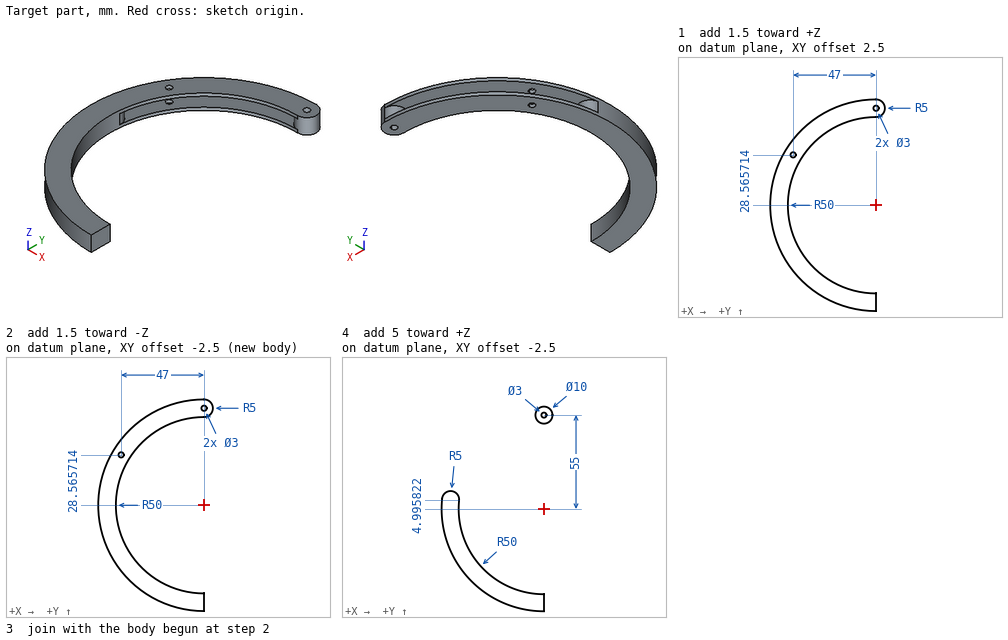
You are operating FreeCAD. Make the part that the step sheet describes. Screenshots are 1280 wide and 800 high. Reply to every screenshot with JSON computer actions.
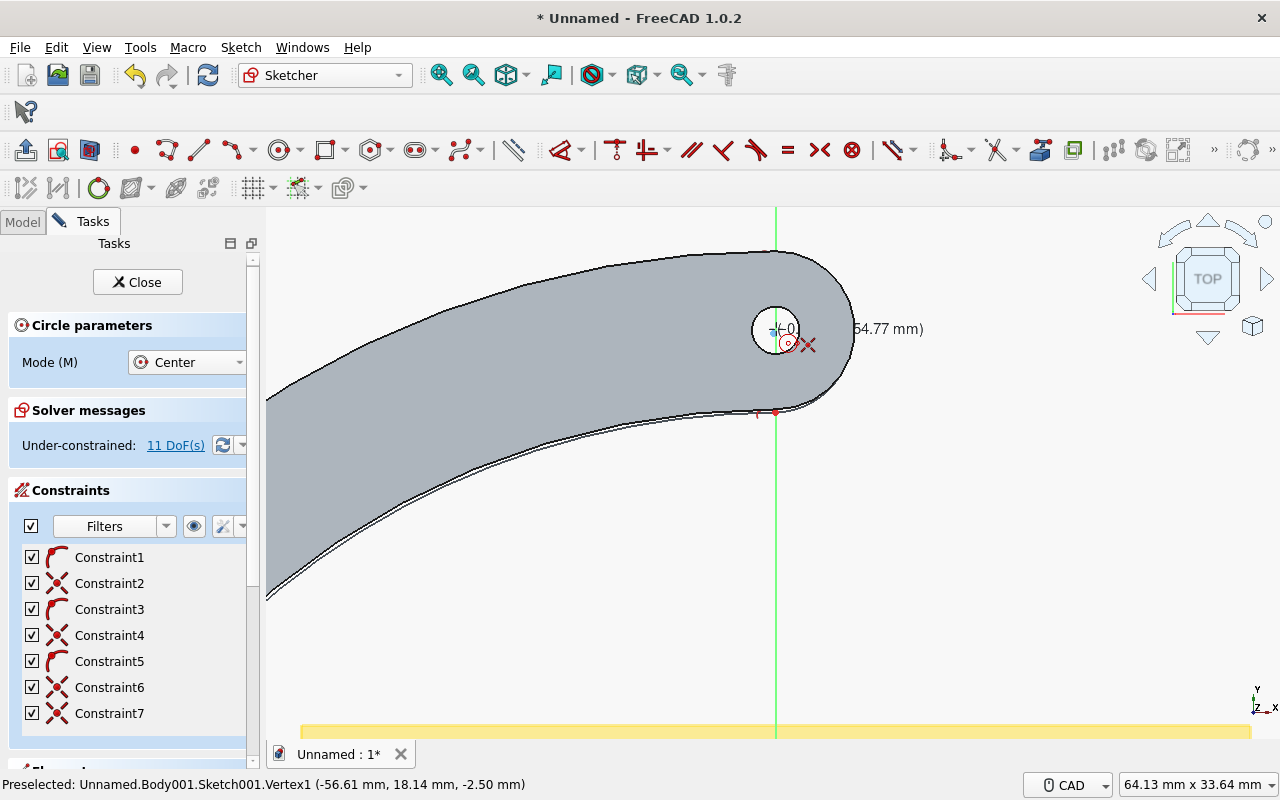
{"action": "scroll", "coordinate": [777, 329], "scroll_direction": "down", "scroll_amount": 9}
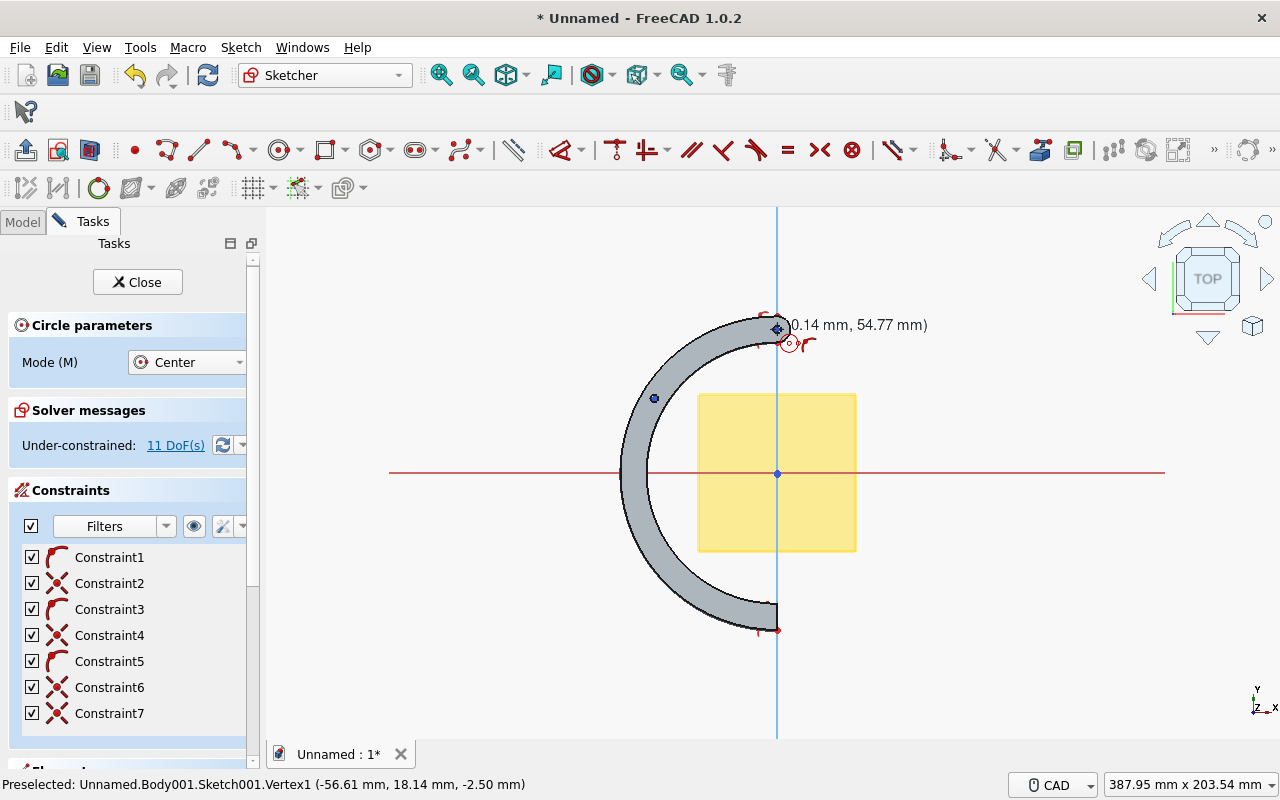
{"action": "left_click", "coordinate": [777, 329]}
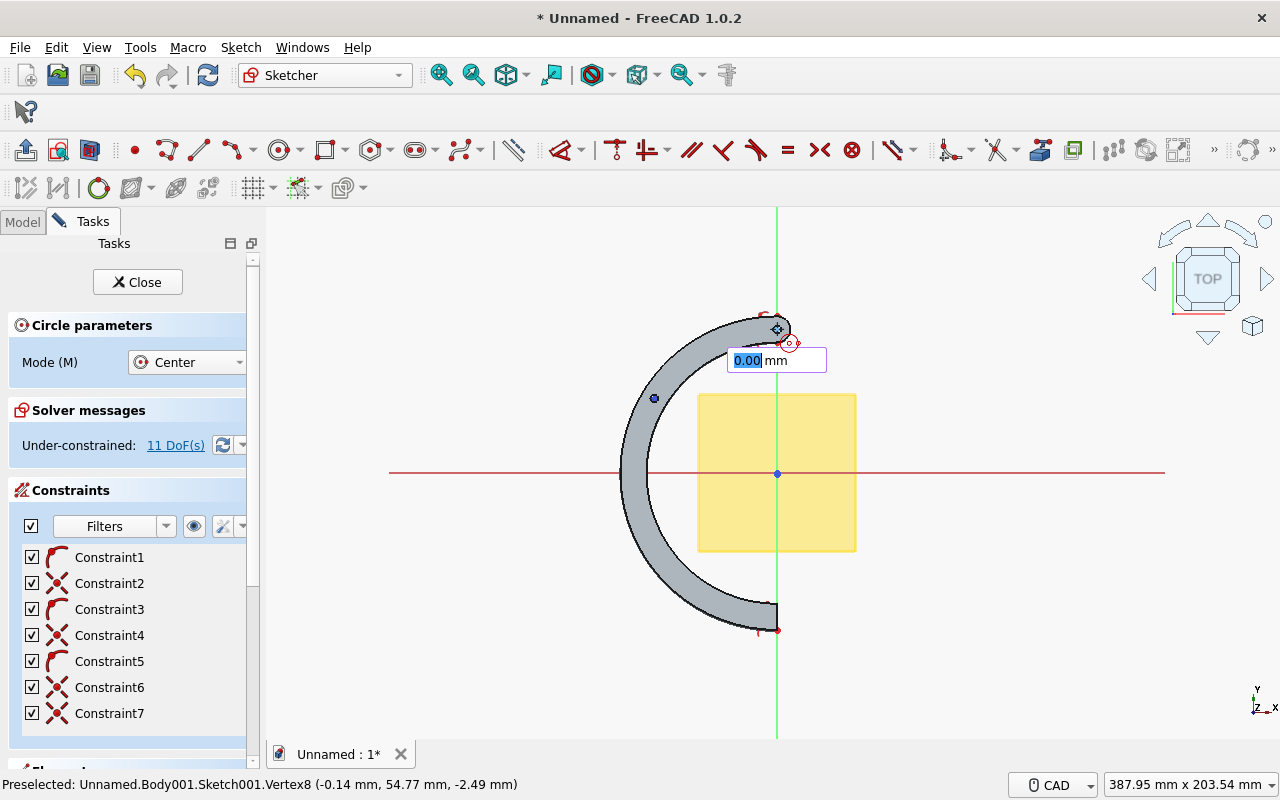
{"action": "scroll", "coordinate": [781, 328], "scroll_direction": "up", "scroll_amount": 8}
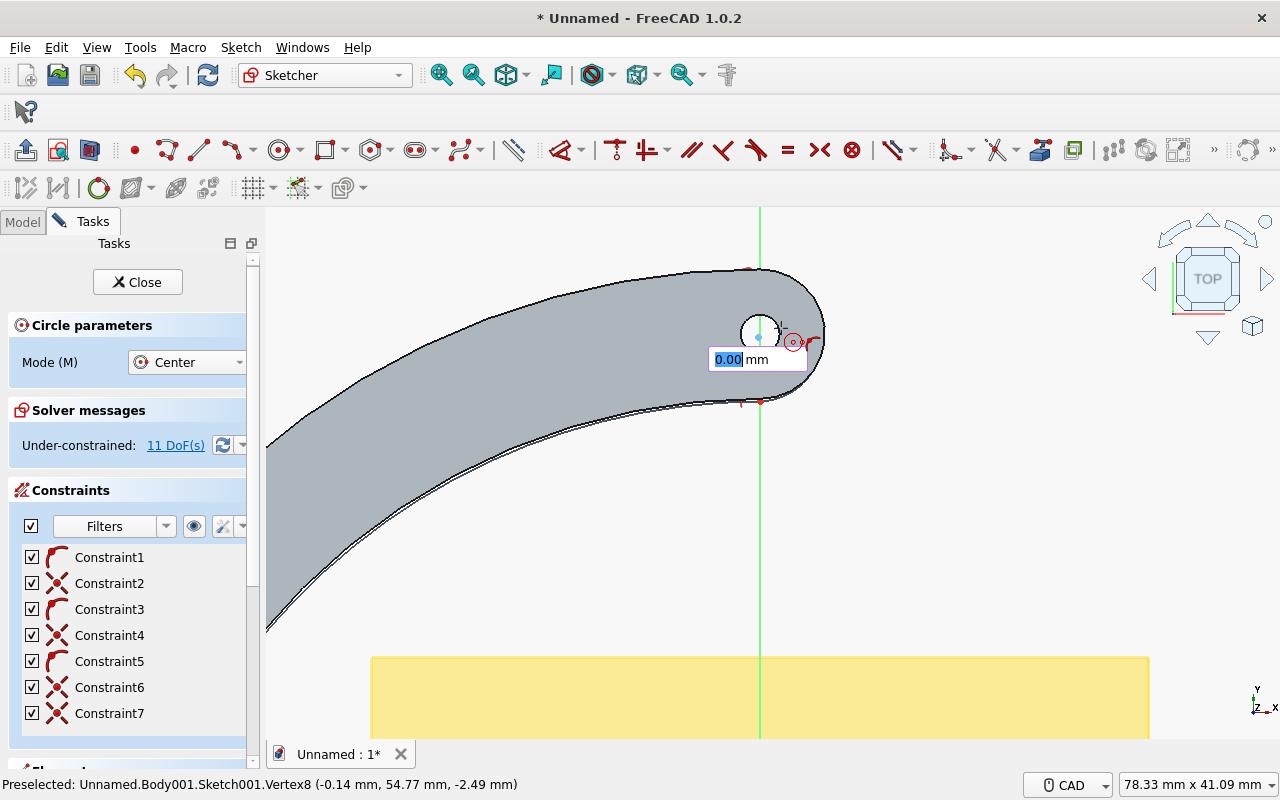
{"action": "left_click", "coordinate": [778, 327]}
{"action": "key", "text": "Escape"}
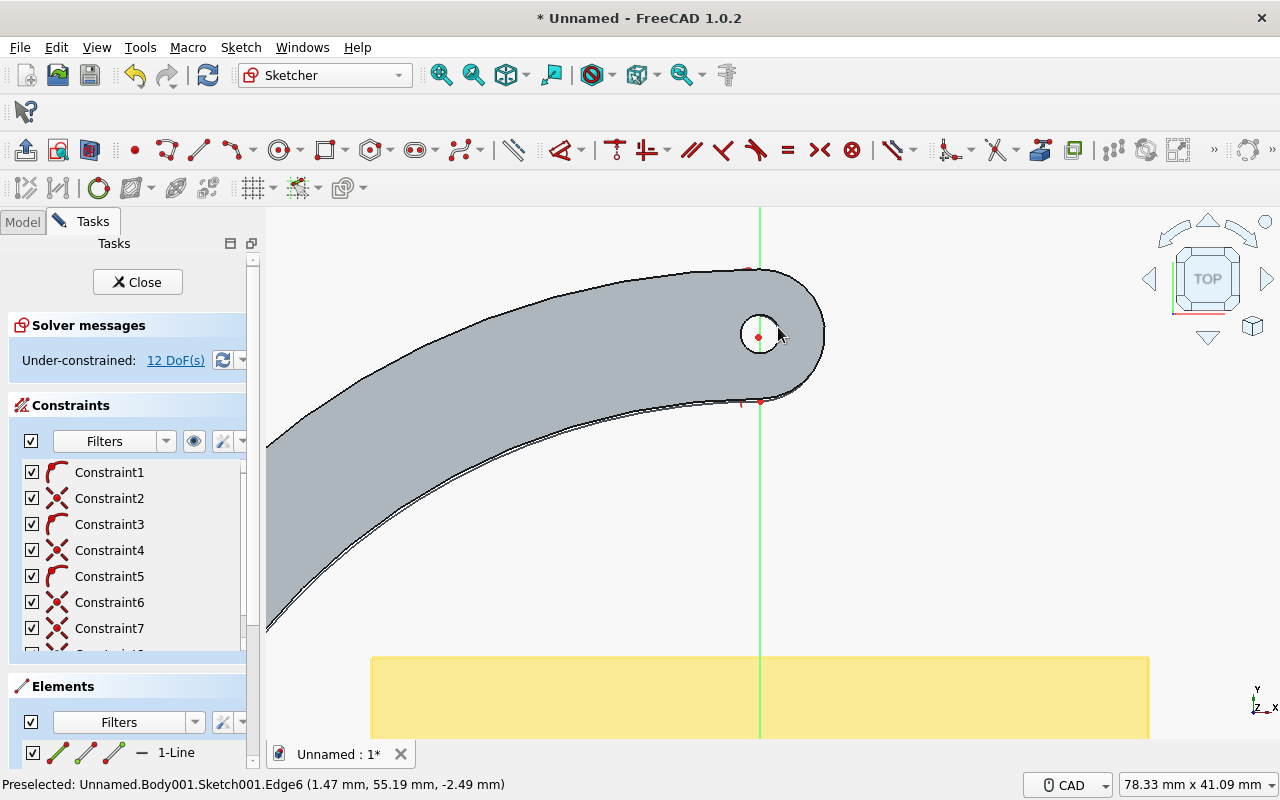
{"action": "scroll", "coordinate": [780, 328], "scroll_direction": "down", "scroll_amount": 8}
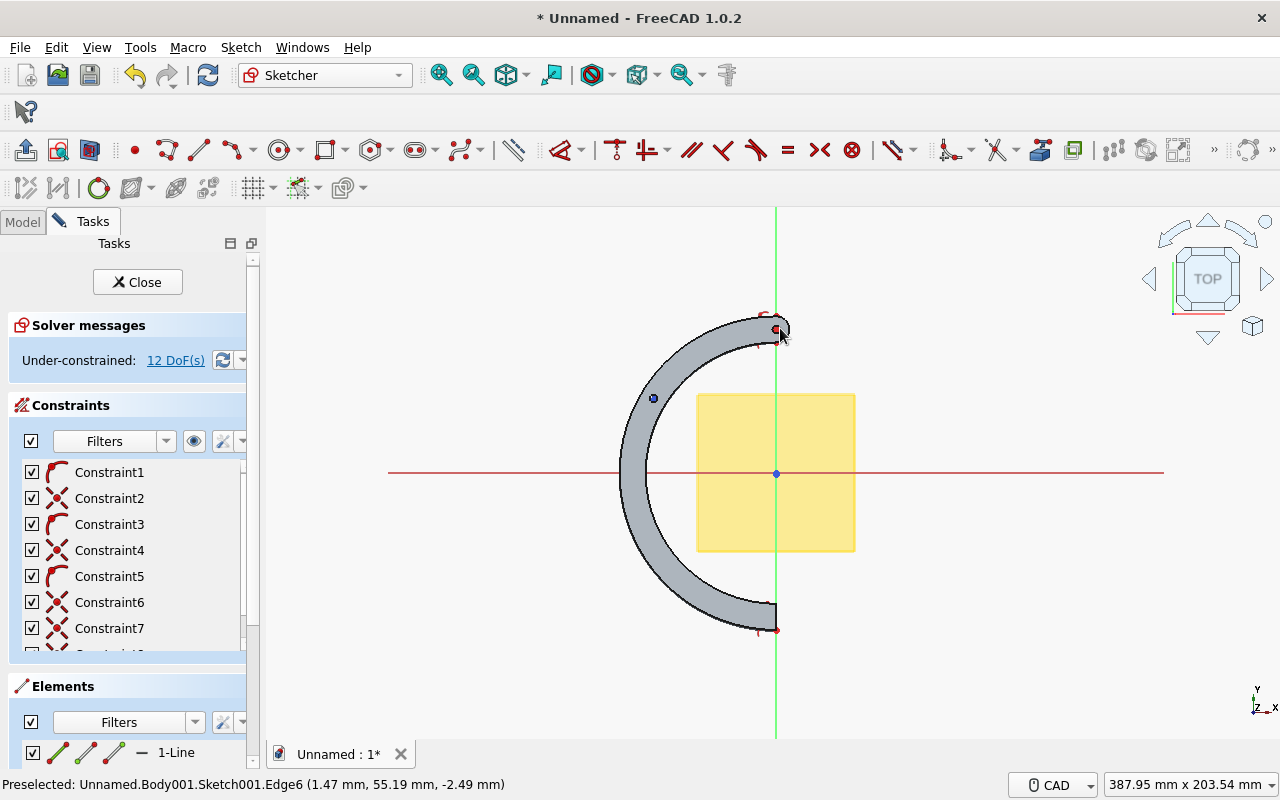
{"action": "left_click", "coordinate": [701, 367]}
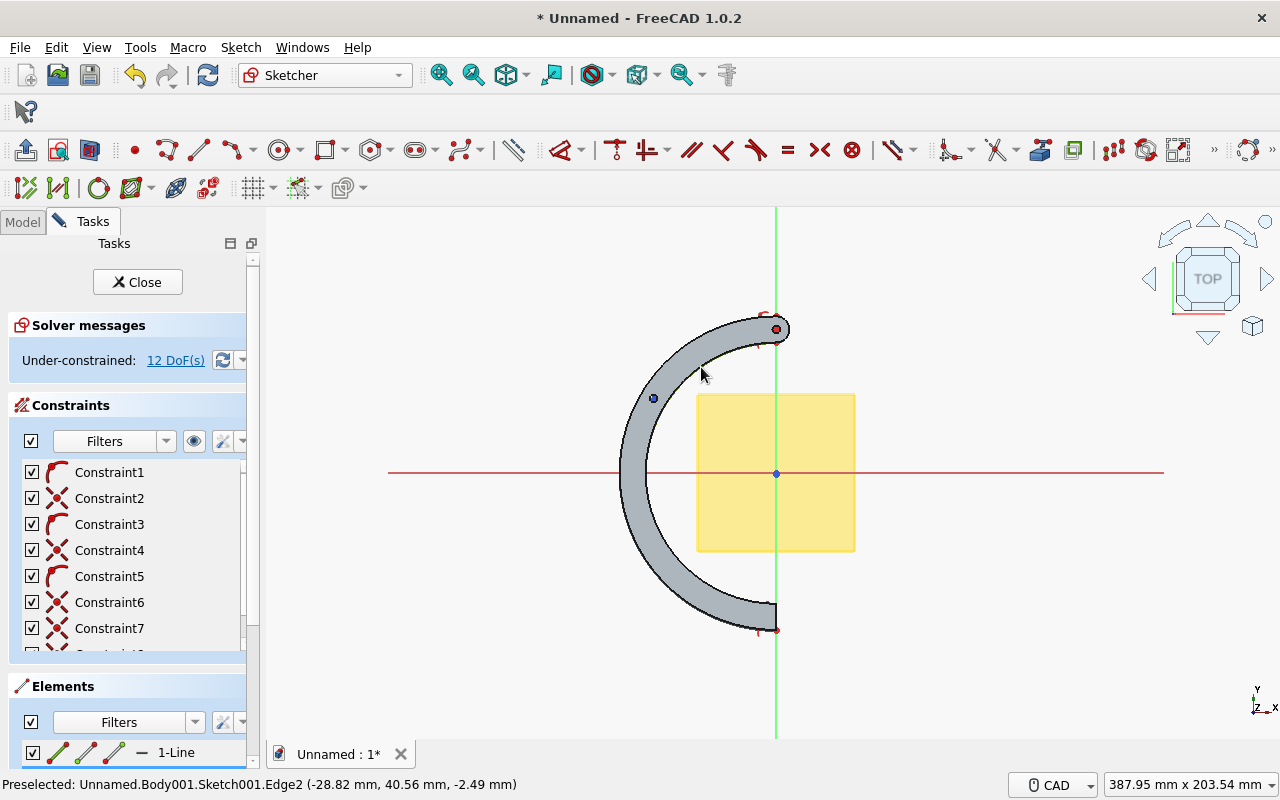
{"action": "scroll", "coordinate": [787, 338], "scroll_direction": "up", "scroll_amount": 3}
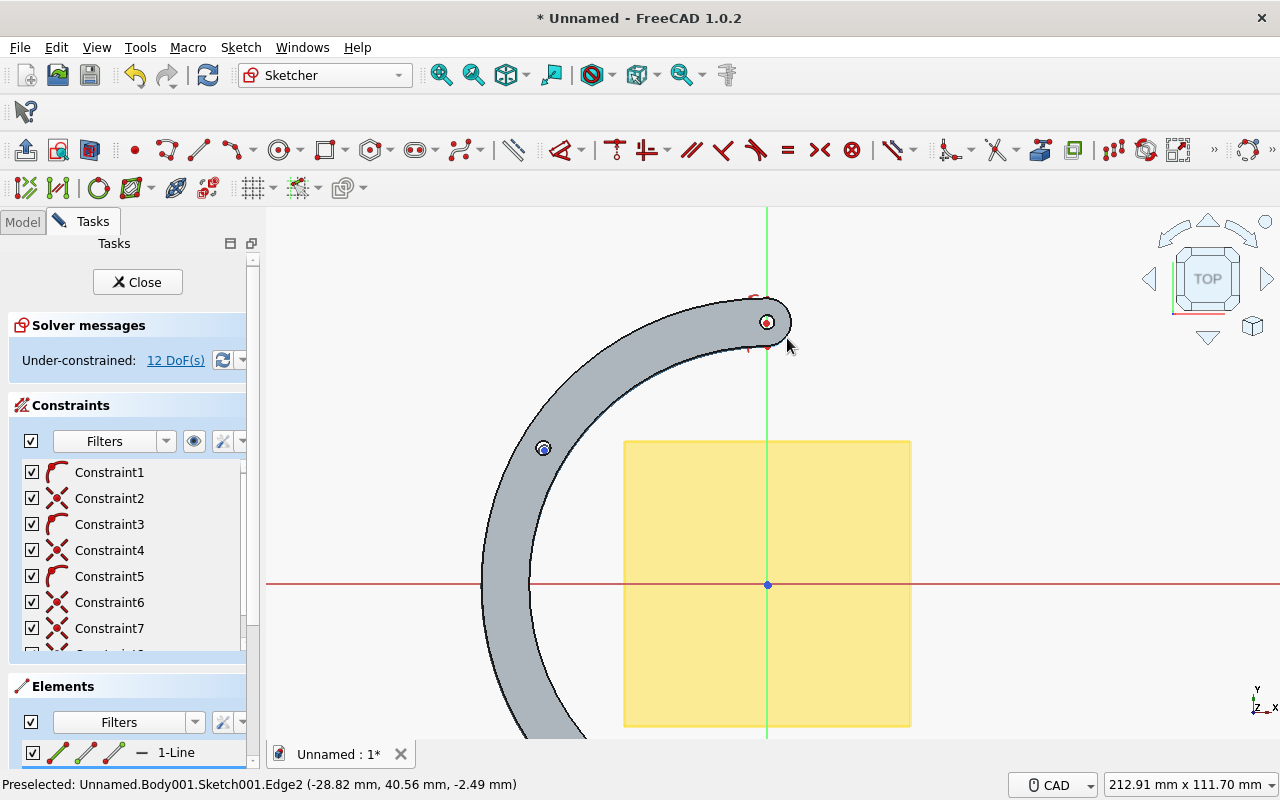
{"action": "left_click", "coordinate": [786, 337]}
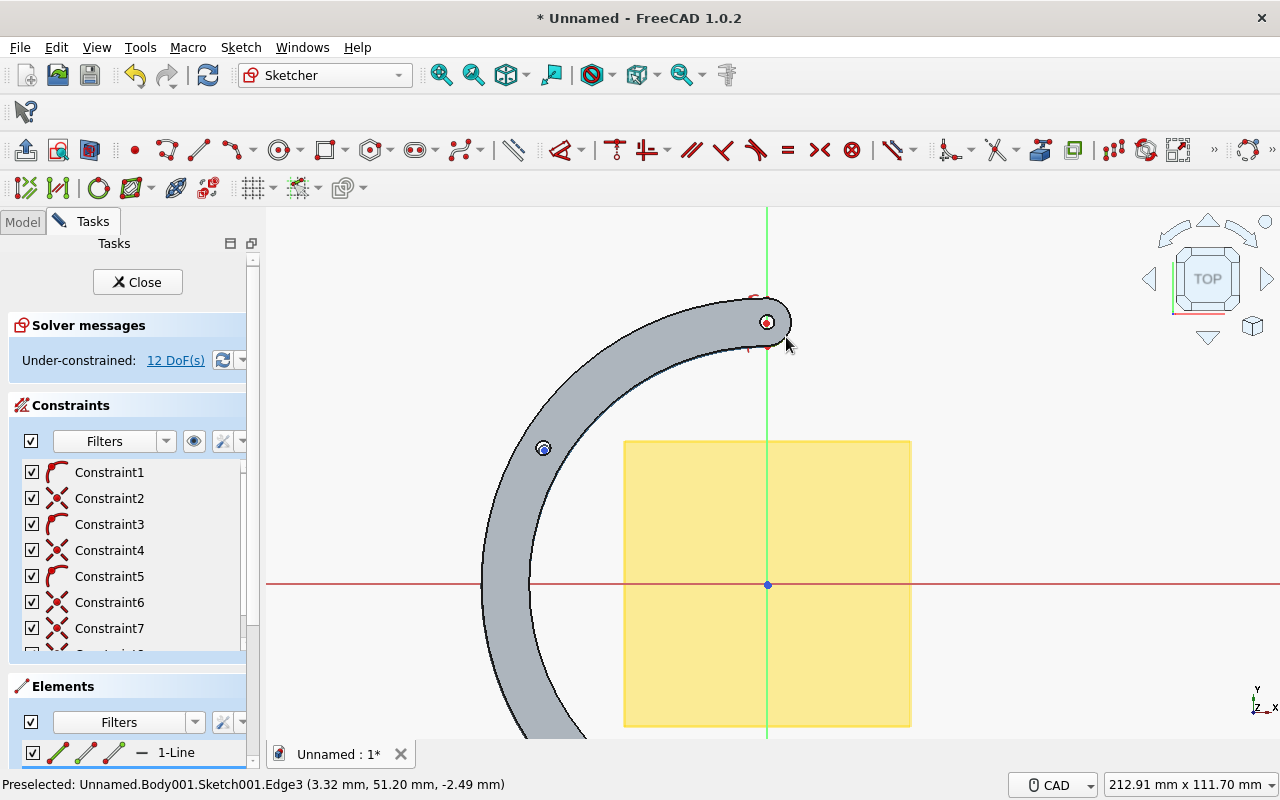
{"action": "left_click", "coordinate": [756, 150]}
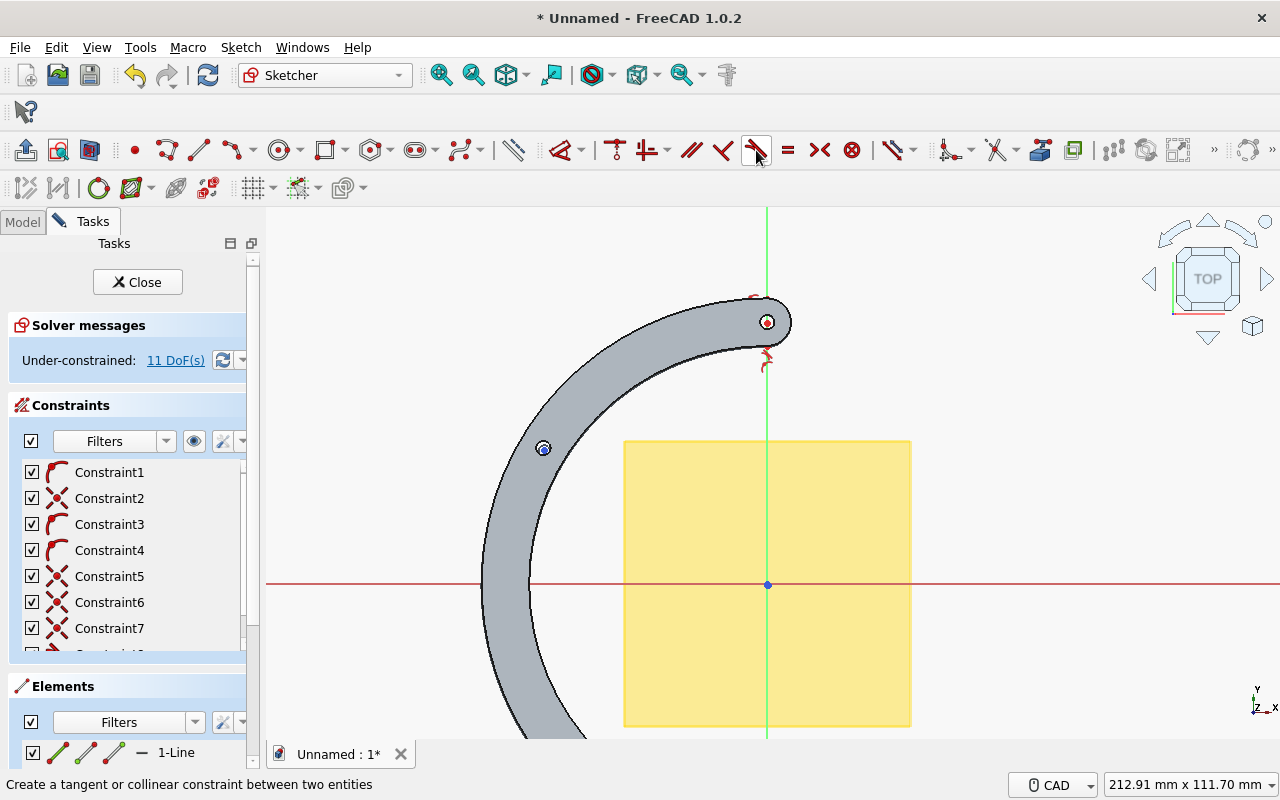
{"action": "scroll", "coordinate": [787, 338], "scroll_direction": "down", "scroll_amount": 3}